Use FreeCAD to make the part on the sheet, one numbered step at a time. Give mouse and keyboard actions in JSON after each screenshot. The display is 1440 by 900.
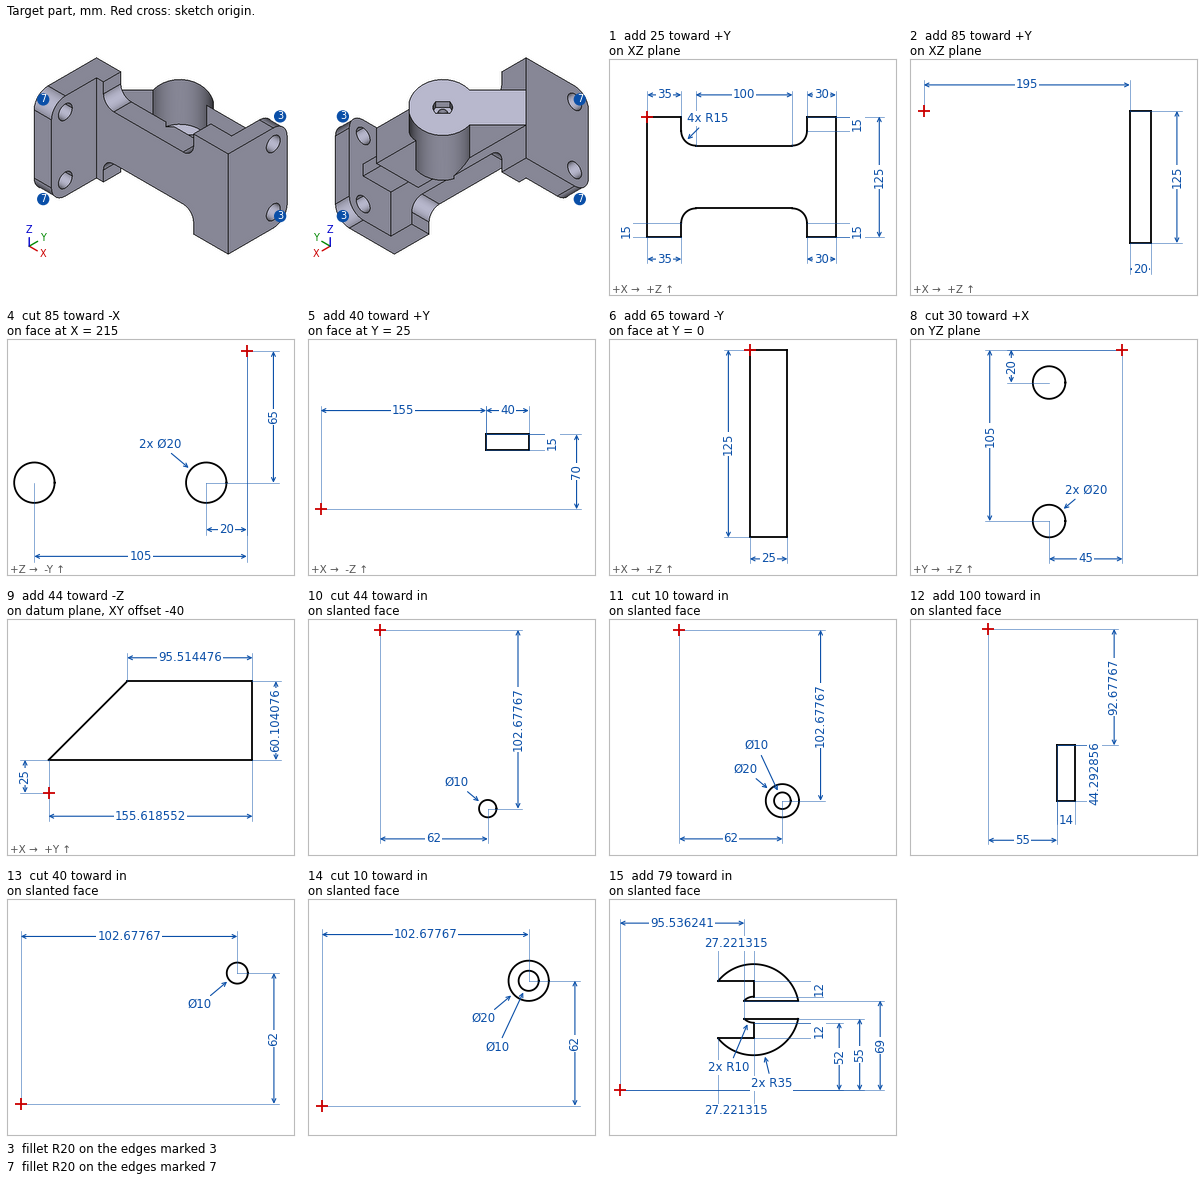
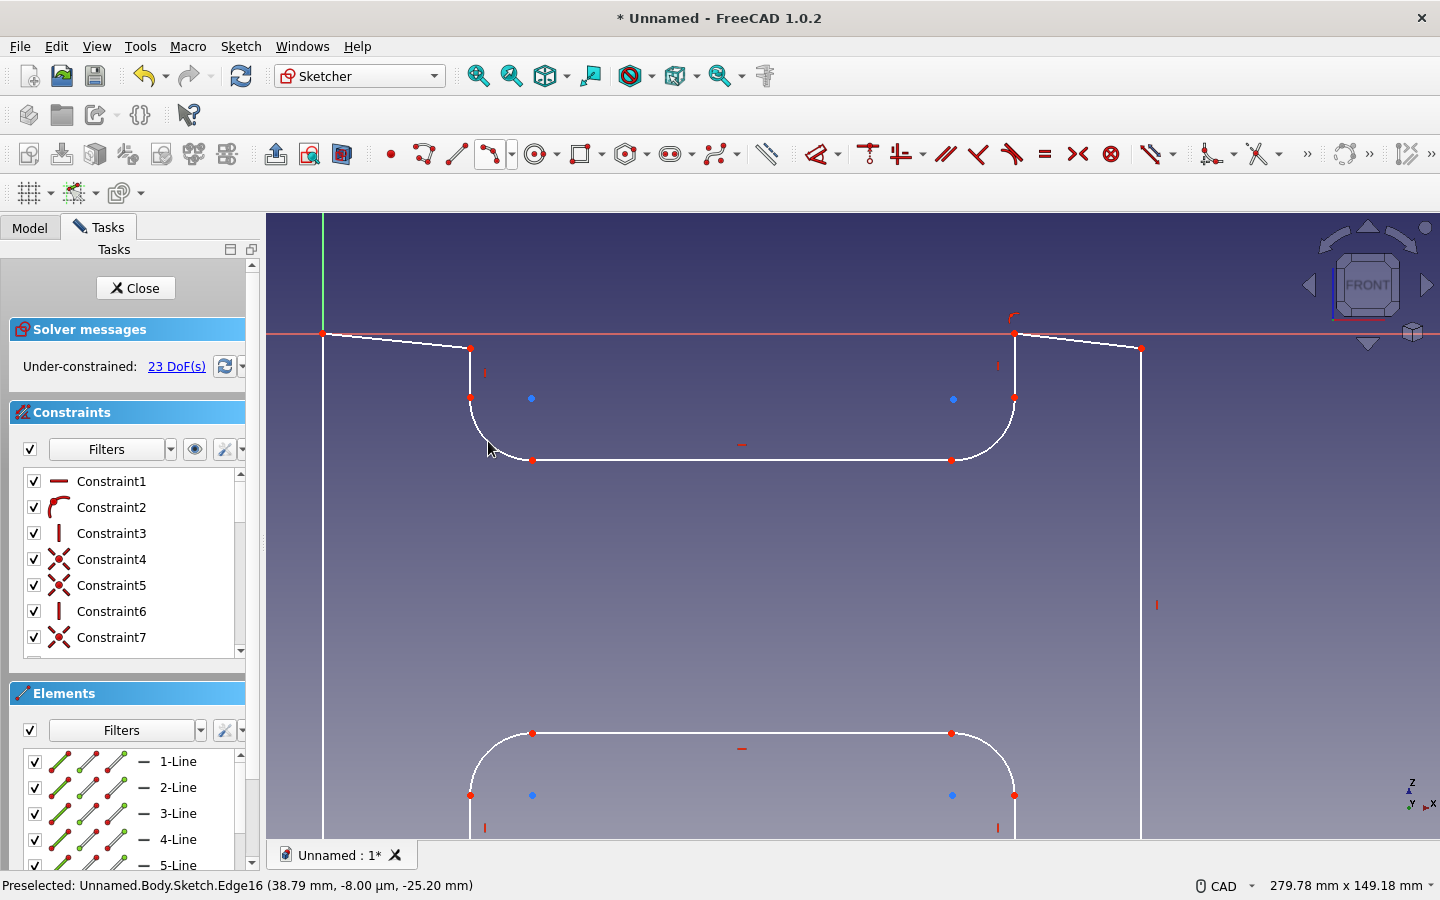
{"action": "left_click", "coordinate": [658, 460]}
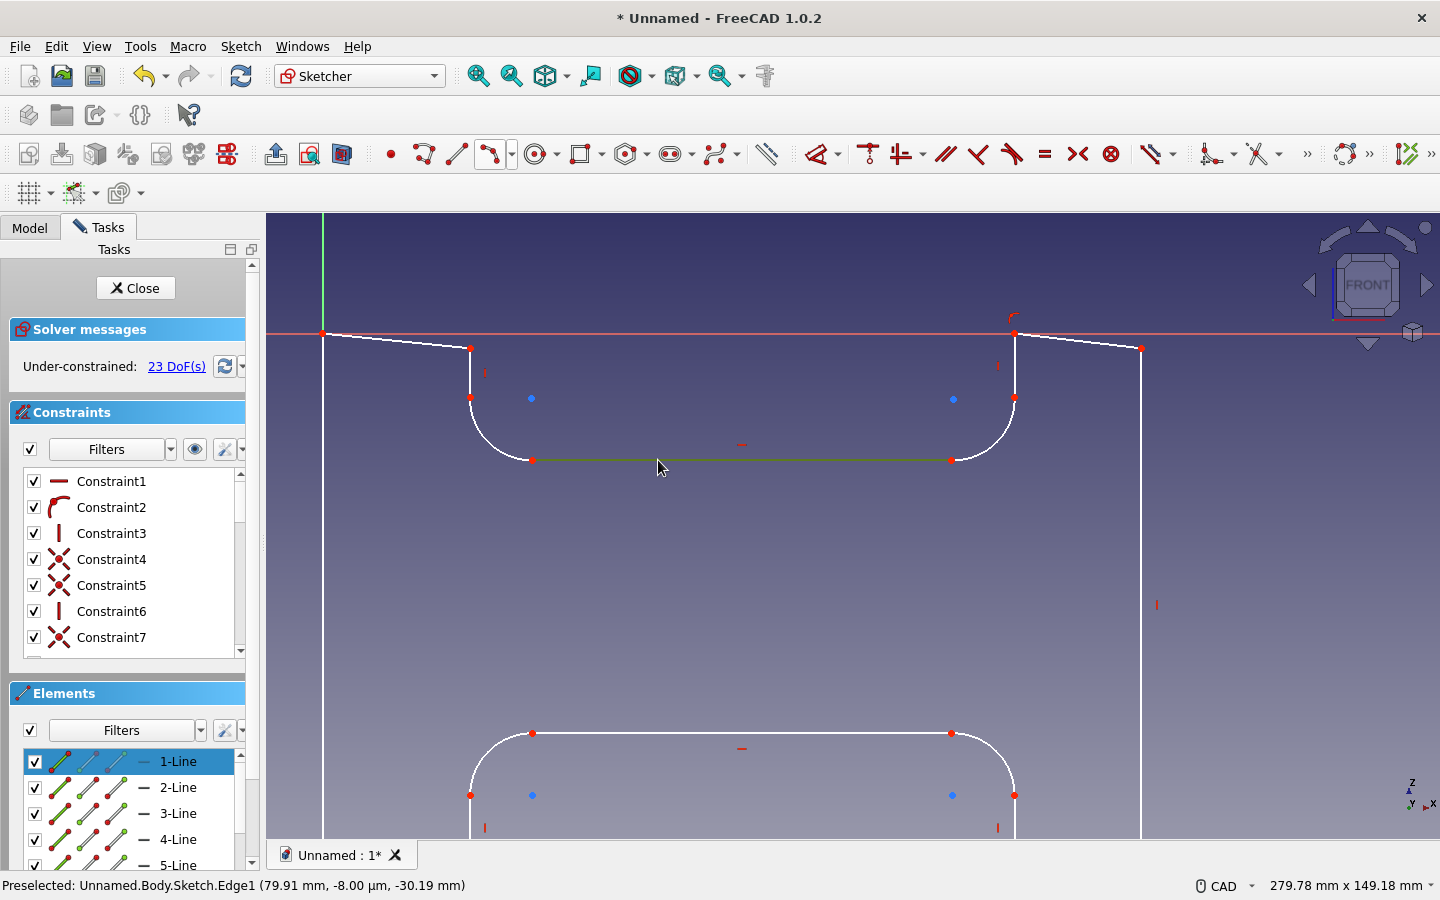
{"action": "left_click", "coordinate": [981, 454]}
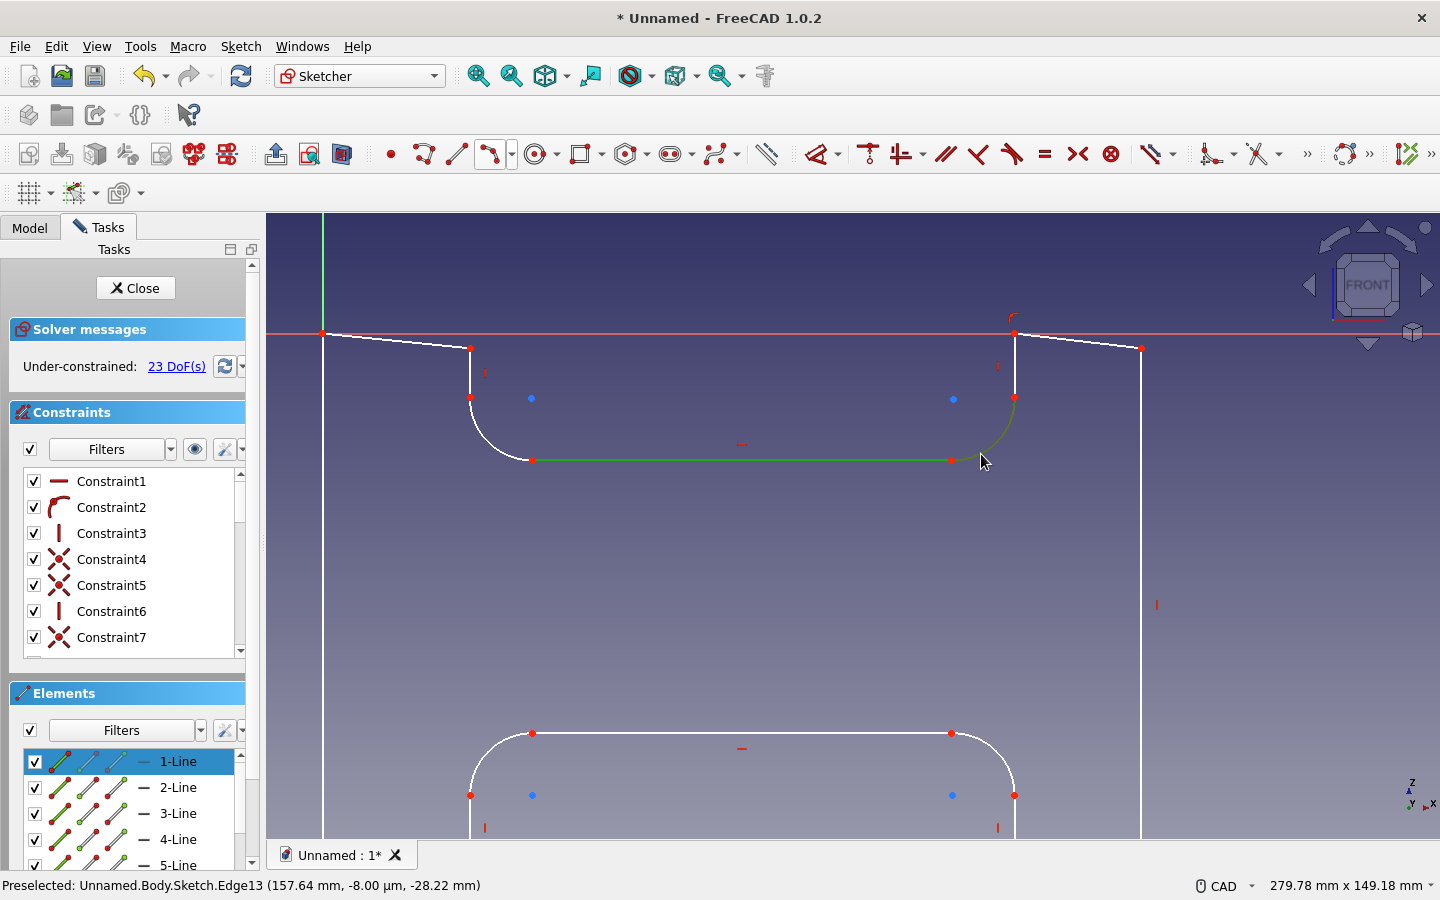
{"action": "key", "text": "t"}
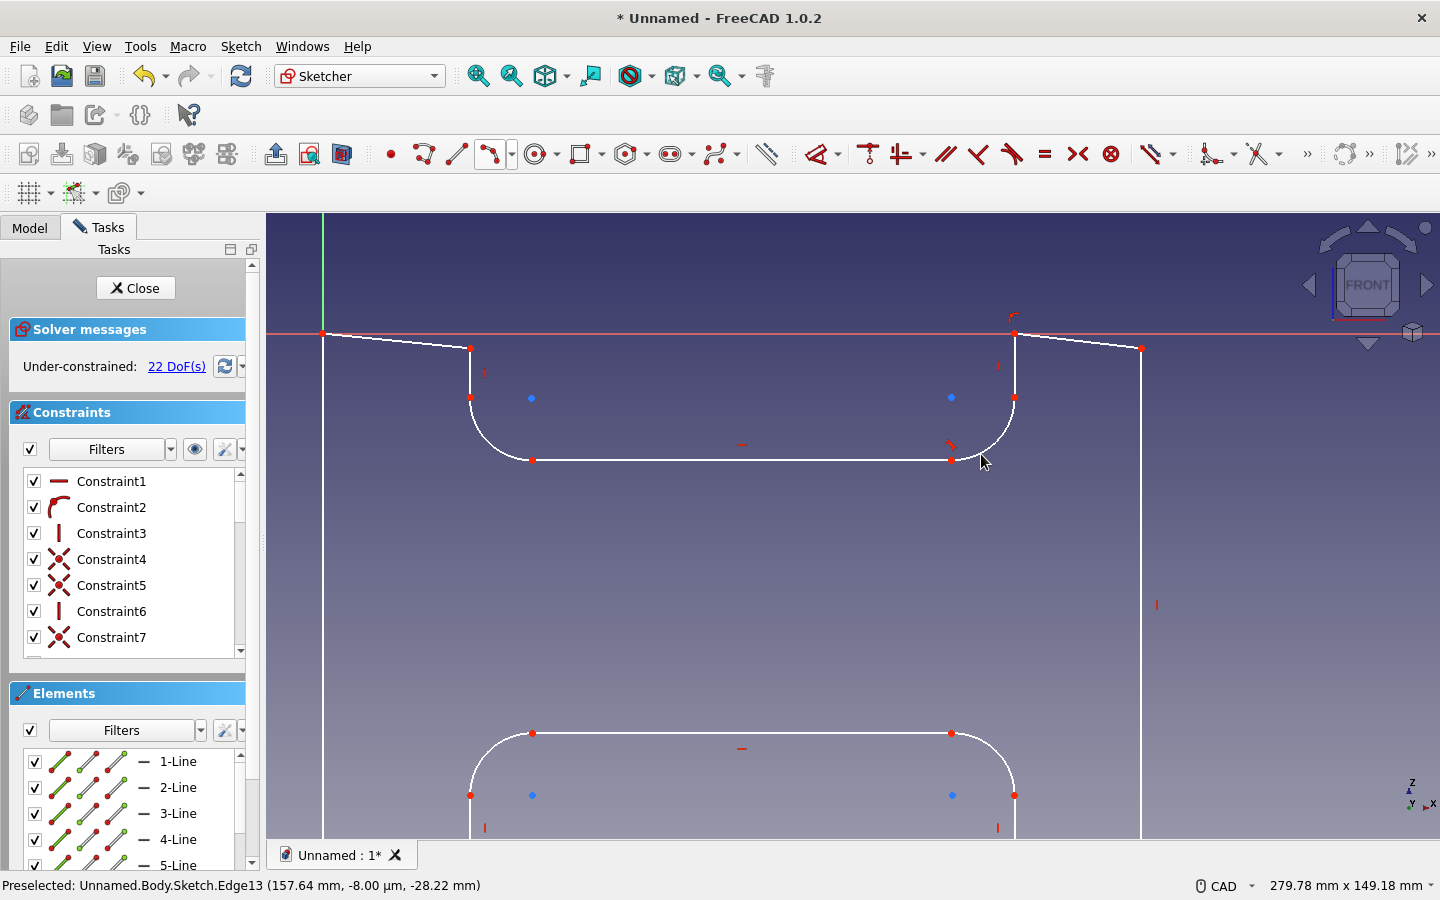
{"action": "left_click", "coordinate": [658, 460]}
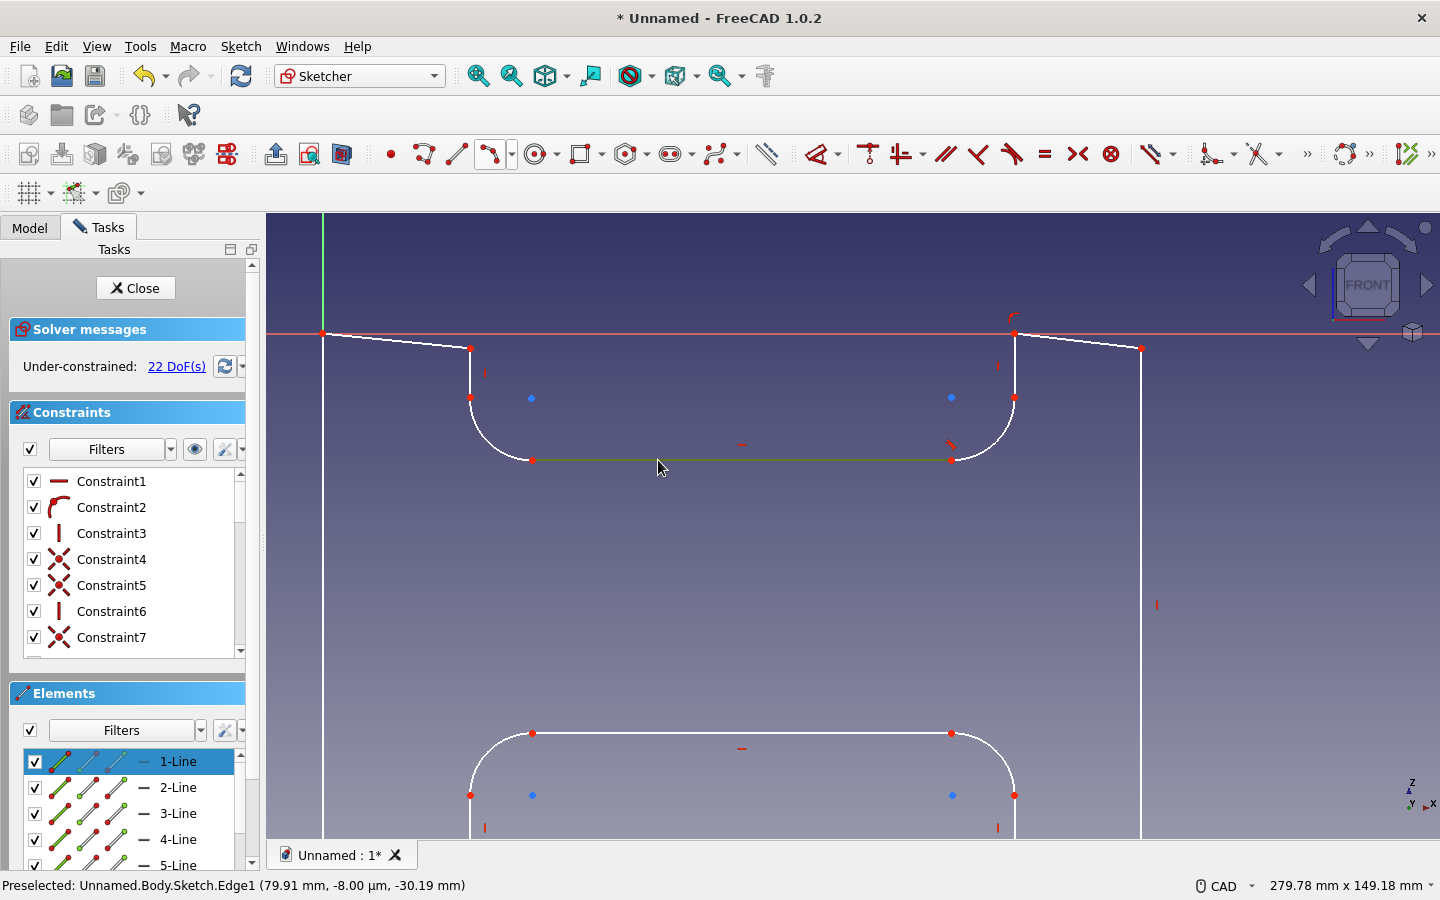
{"action": "left_click", "coordinate": [477, 426]}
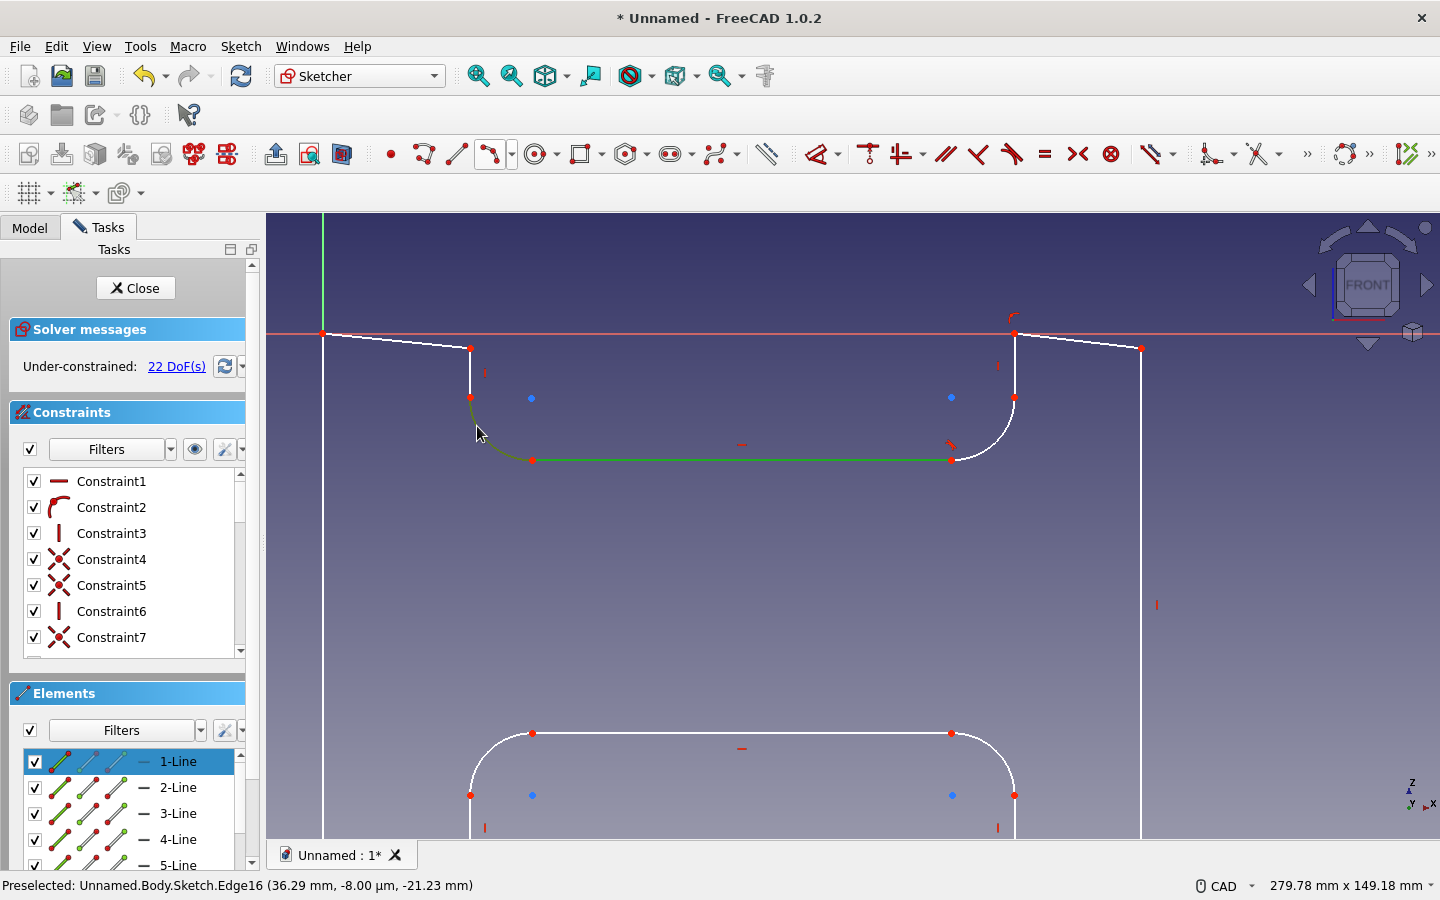
{"action": "left_click", "coordinate": [1012, 154]}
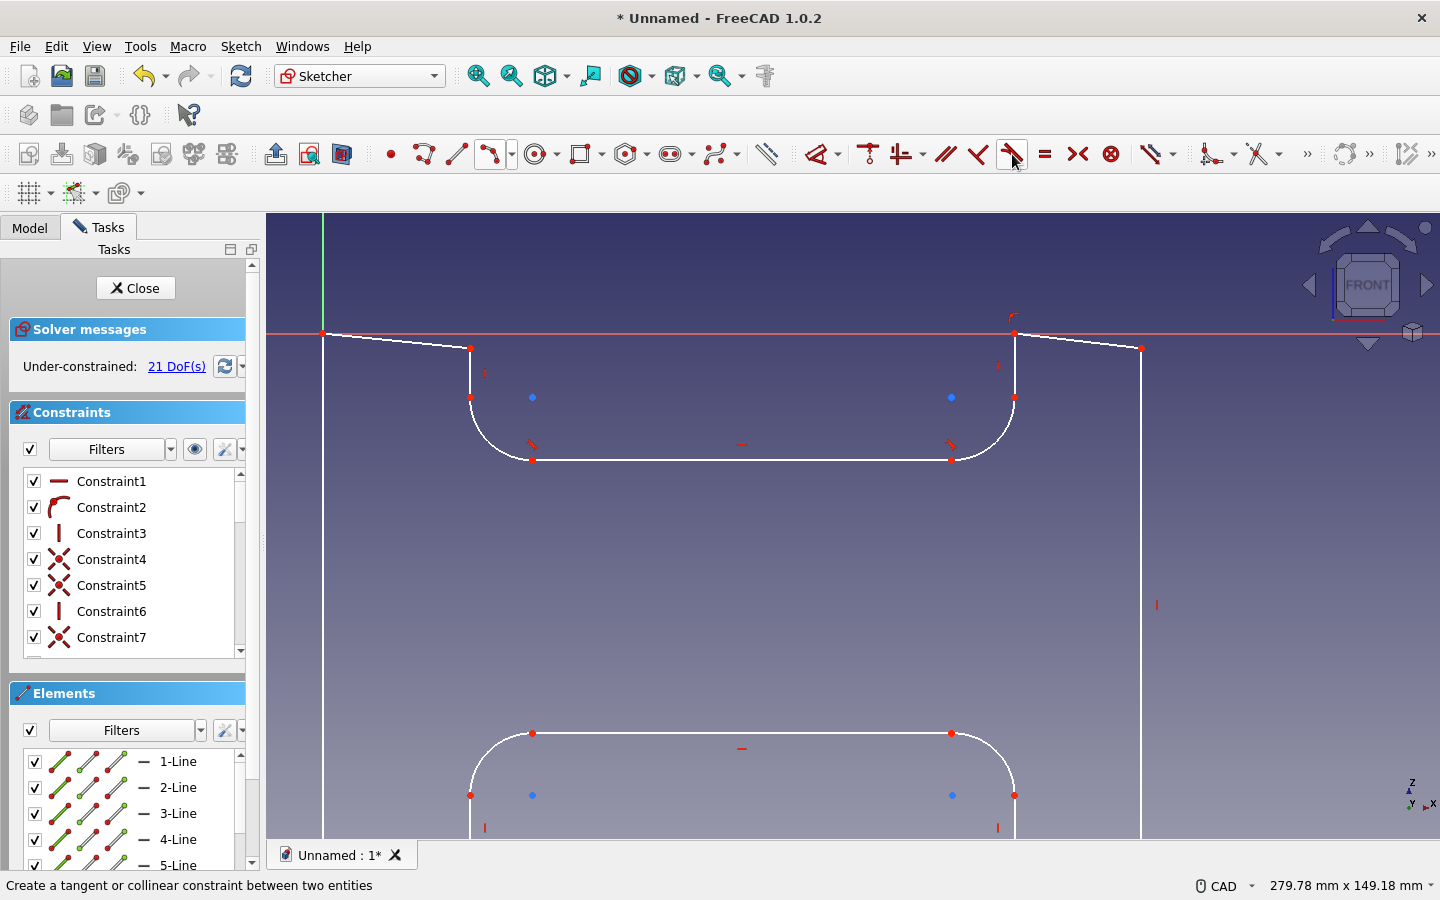
{"action": "left_click", "coordinate": [1015, 378]}